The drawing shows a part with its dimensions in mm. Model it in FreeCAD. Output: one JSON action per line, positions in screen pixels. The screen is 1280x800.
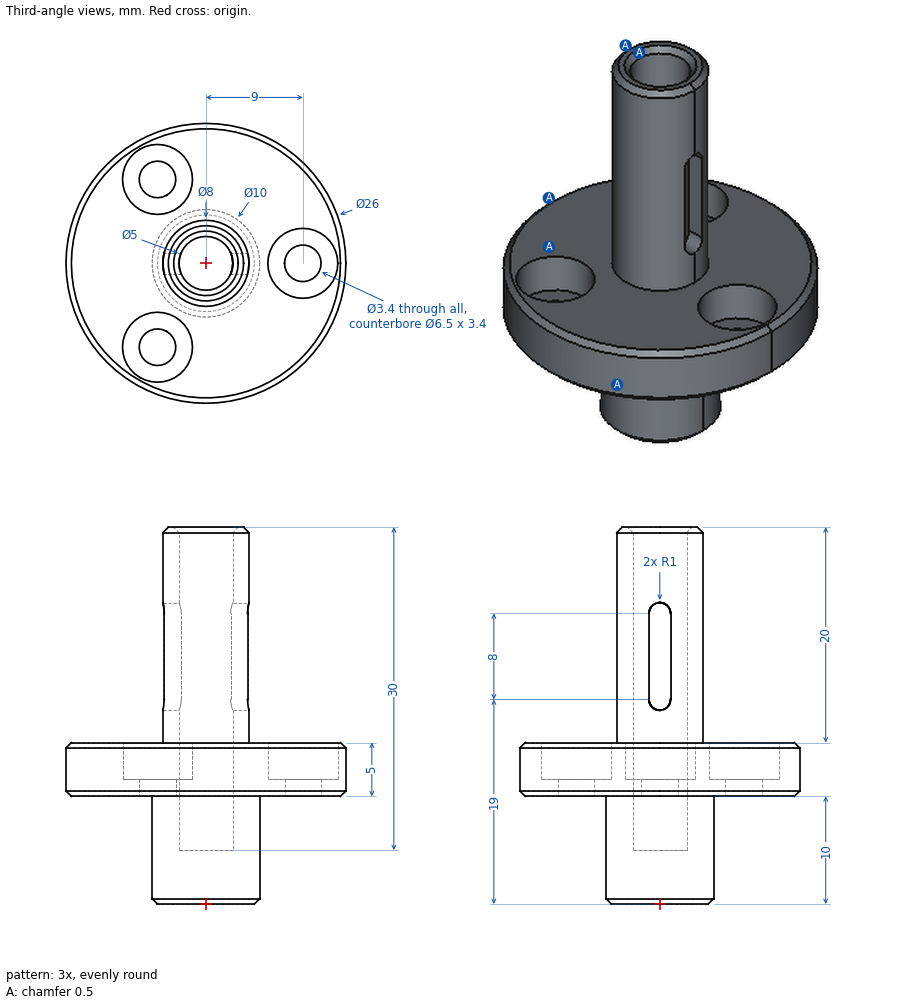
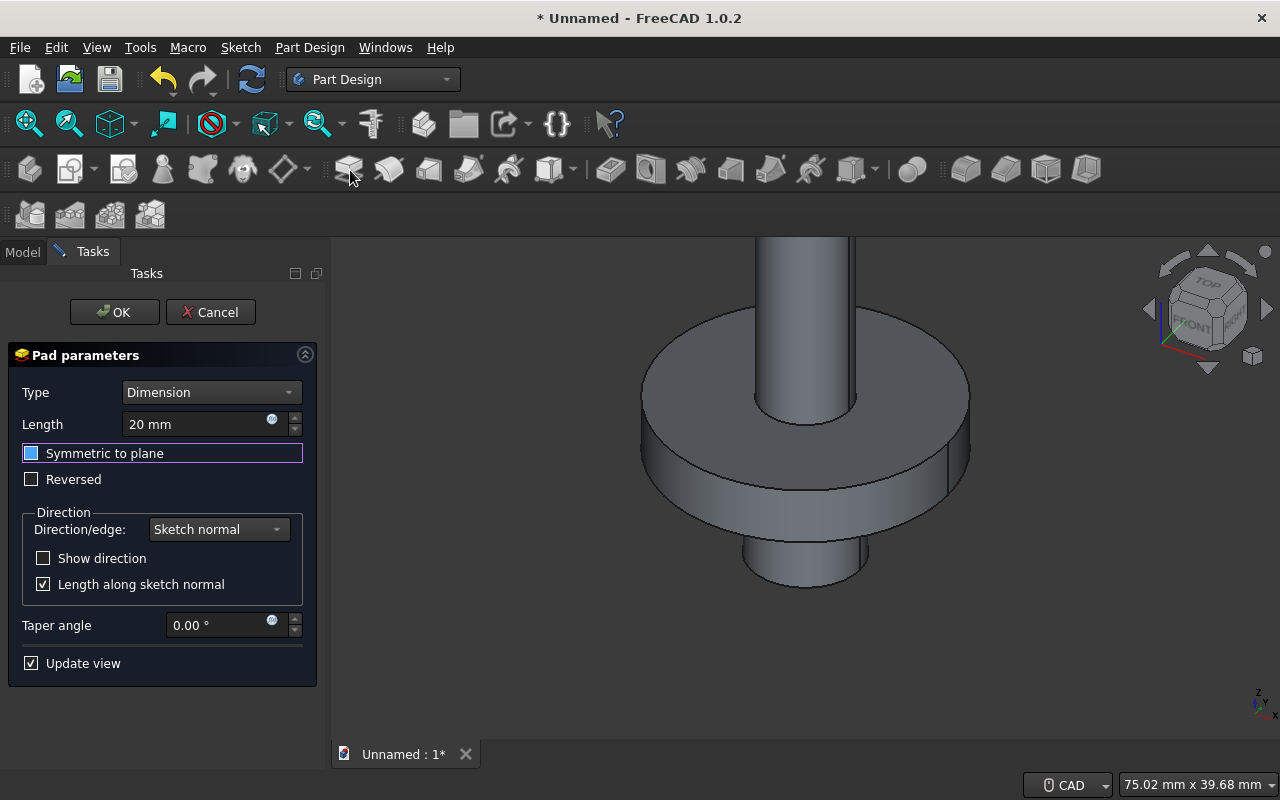
{"action": "left_click", "coordinate": [115, 312]}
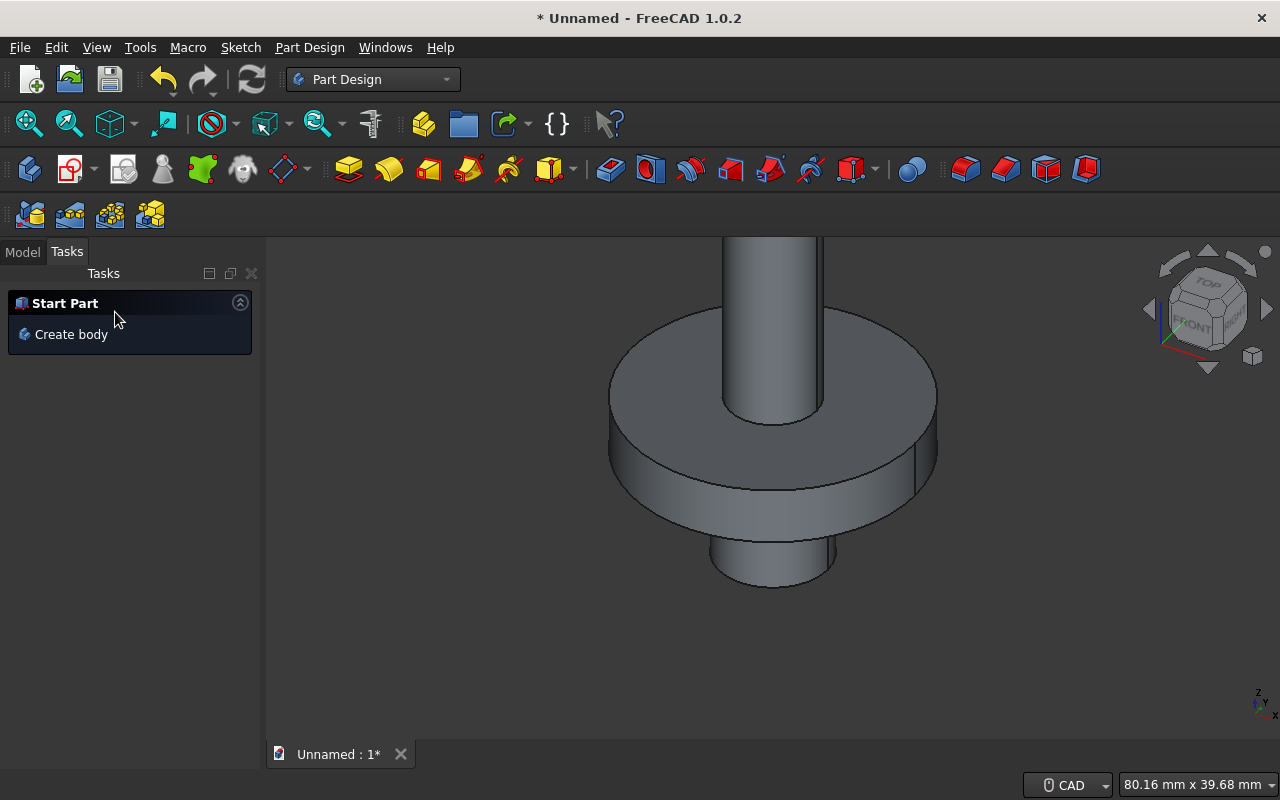
{"action": "left_click", "coordinate": [30, 124]}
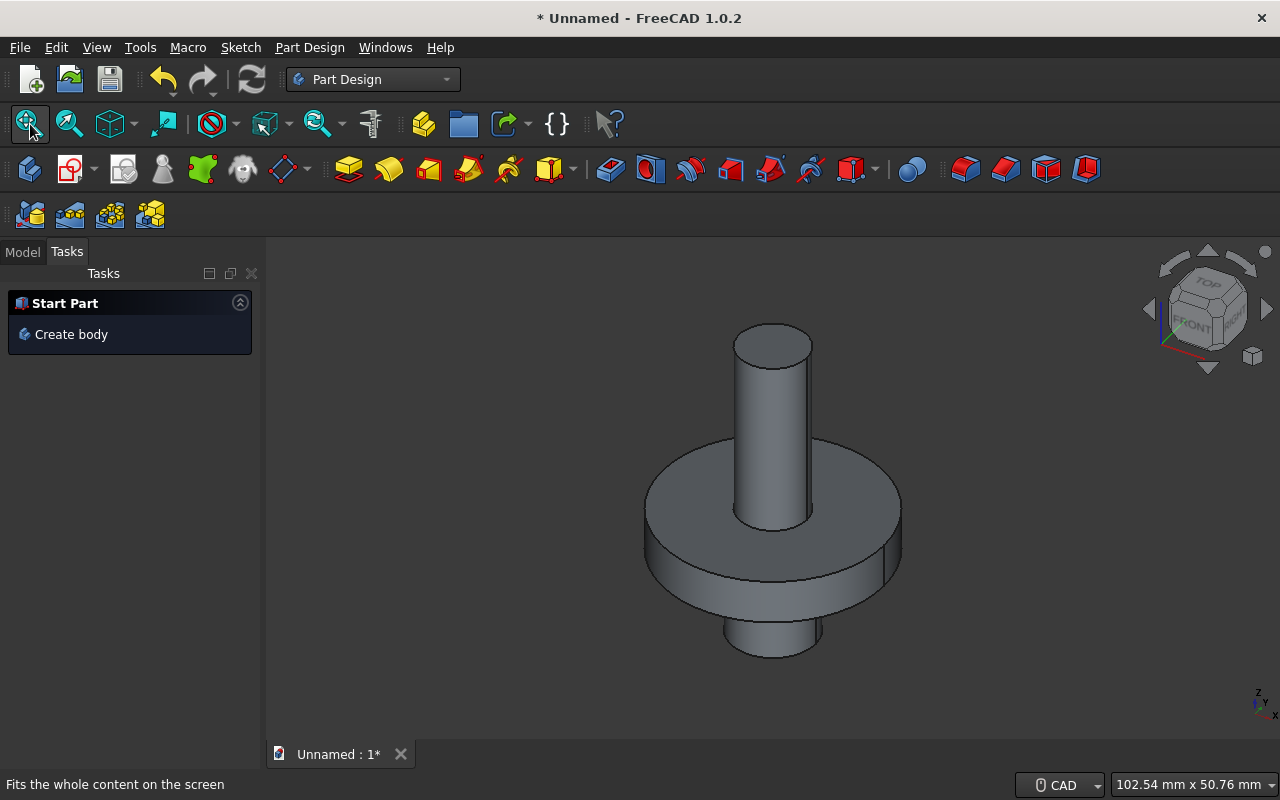
{"action": "left_click", "coordinate": [773, 345]}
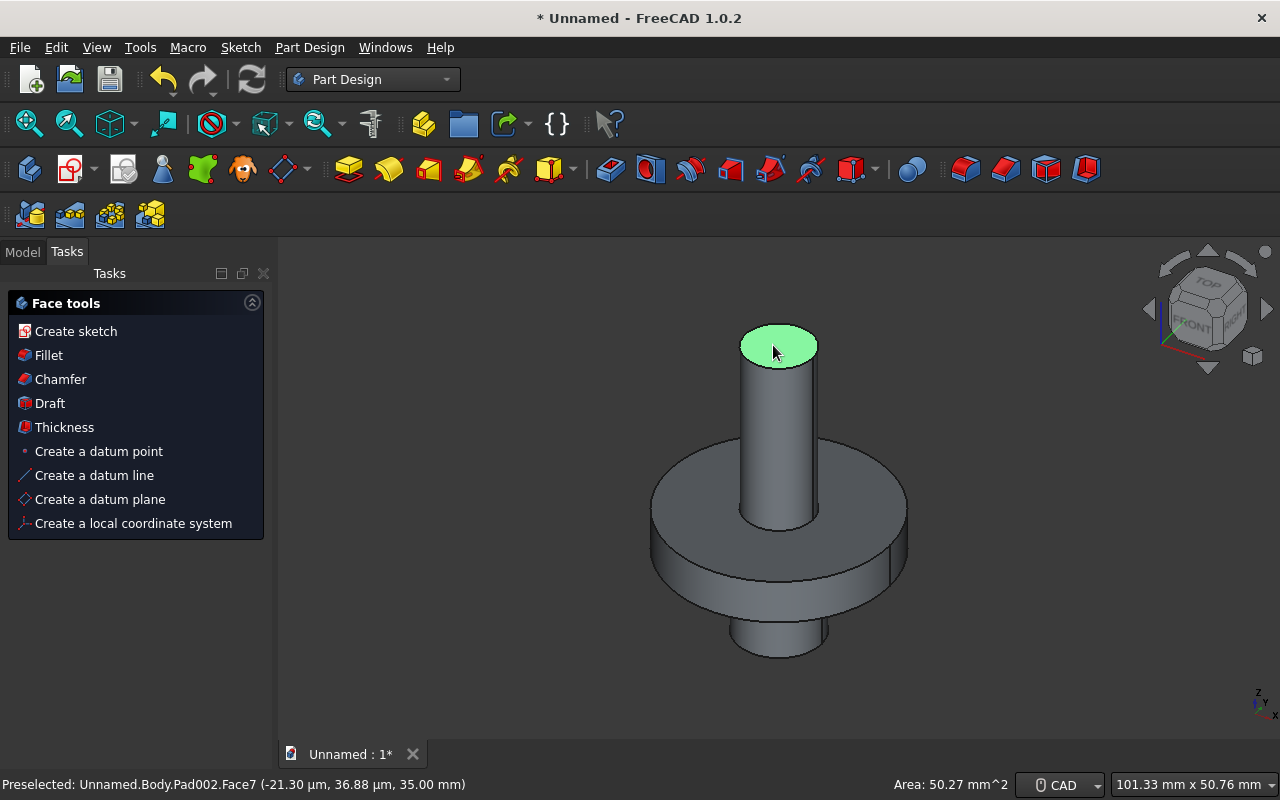
{"action": "left_click", "coordinate": [70, 170]}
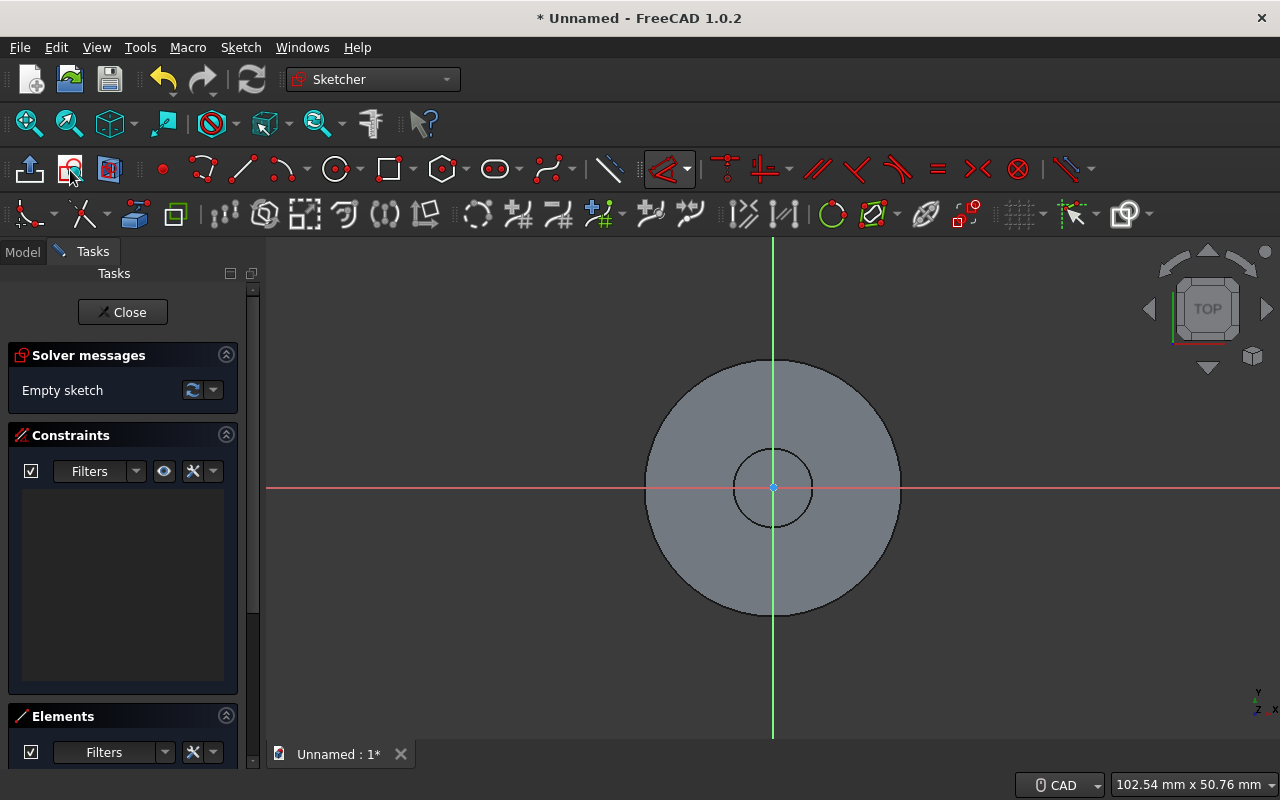
{"action": "scroll", "coordinate": [787, 488], "scroll_direction": "up", "scroll_amount": 9}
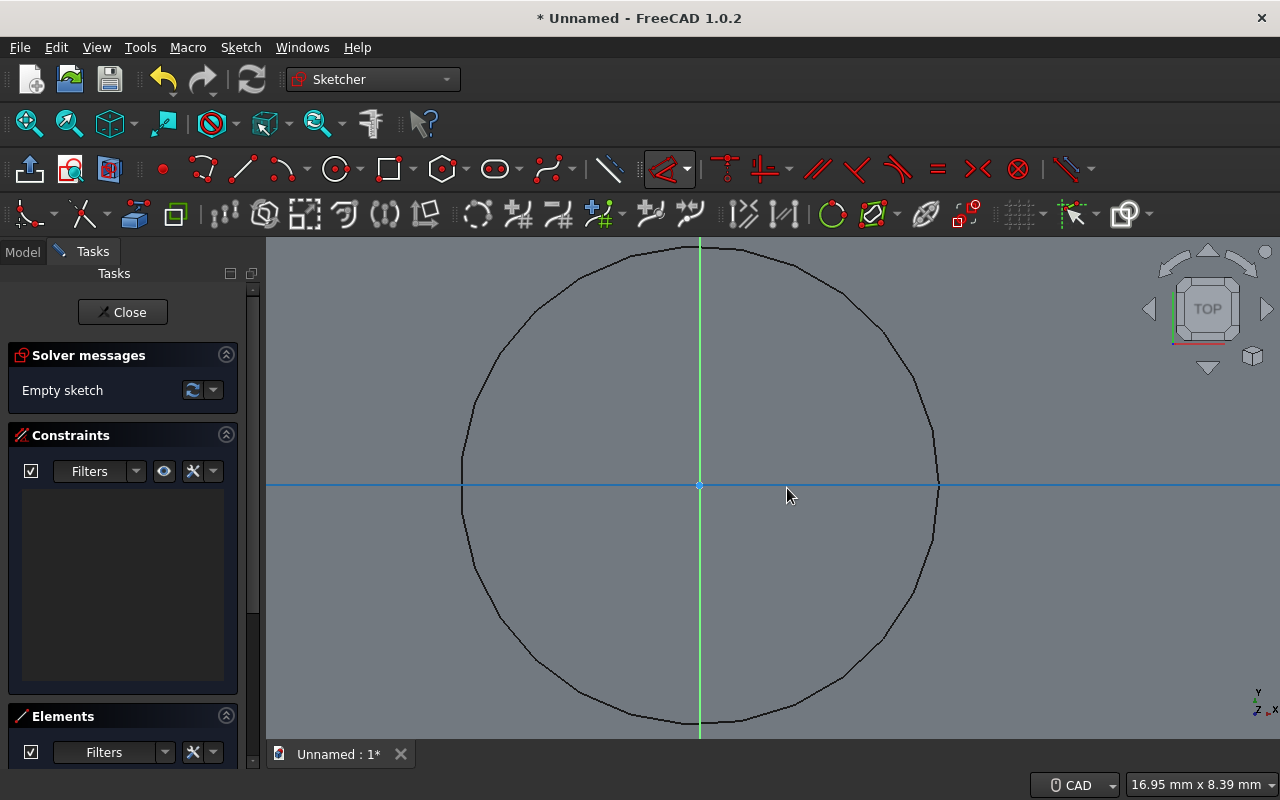
{"action": "left_click", "coordinate": [336, 170]}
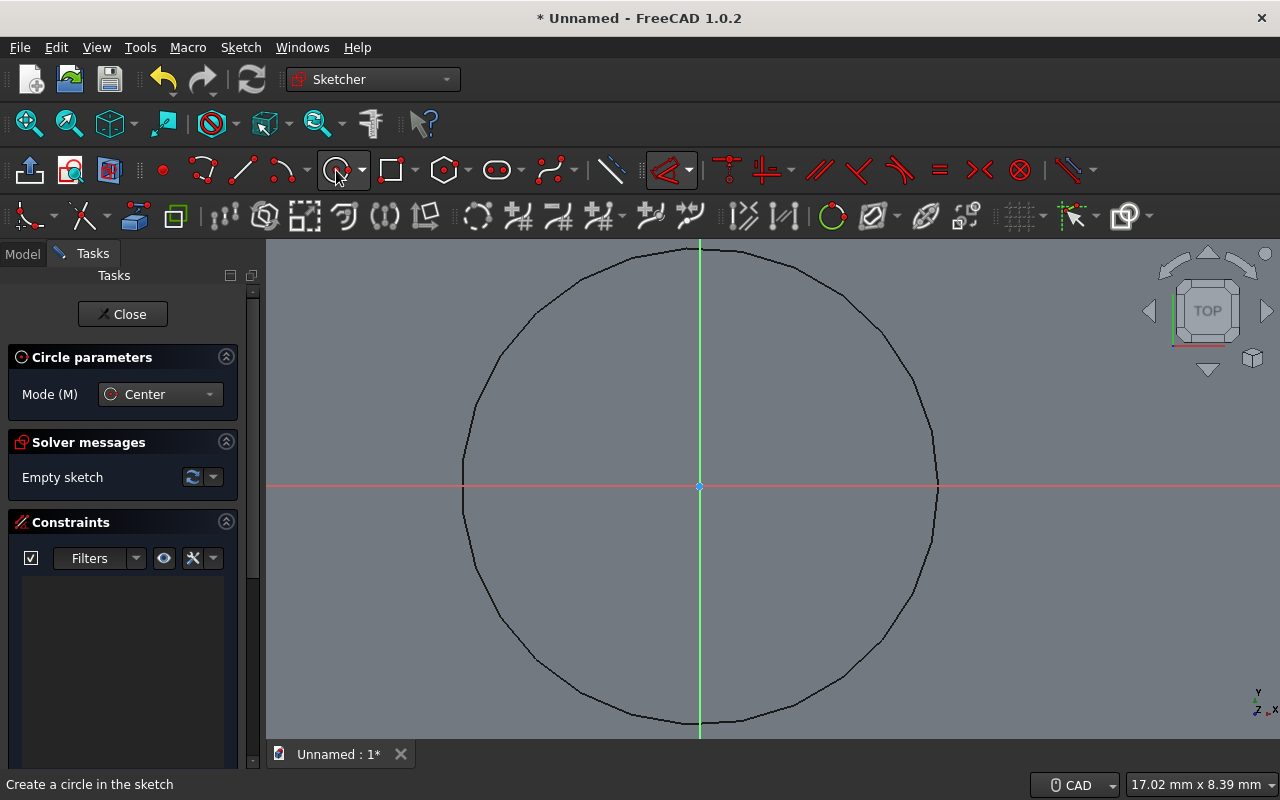
{"action": "left_click", "coordinate": [700, 486]}
{"action": "left_click", "coordinate": [805, 381]}
{"action": "key", "text": "Escape"}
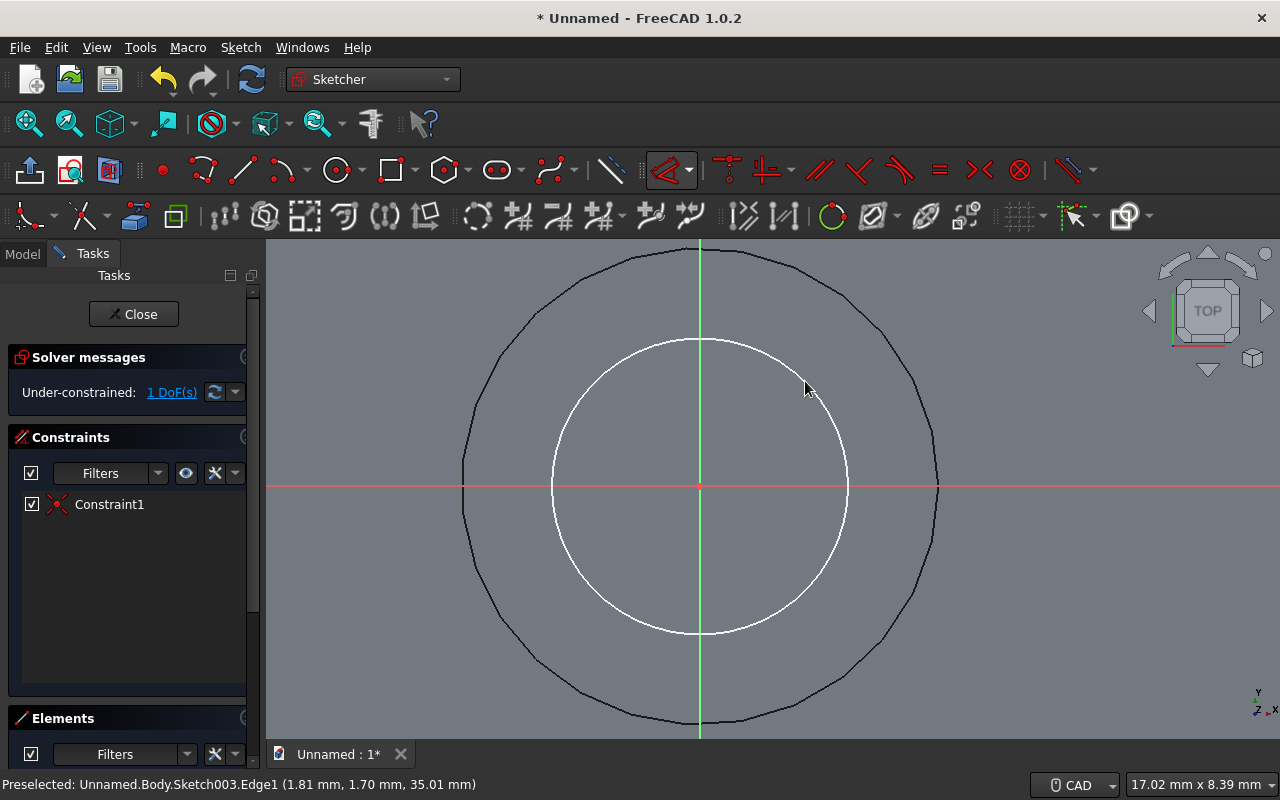
{"action": "left_click", "coordinate": [804, 381]}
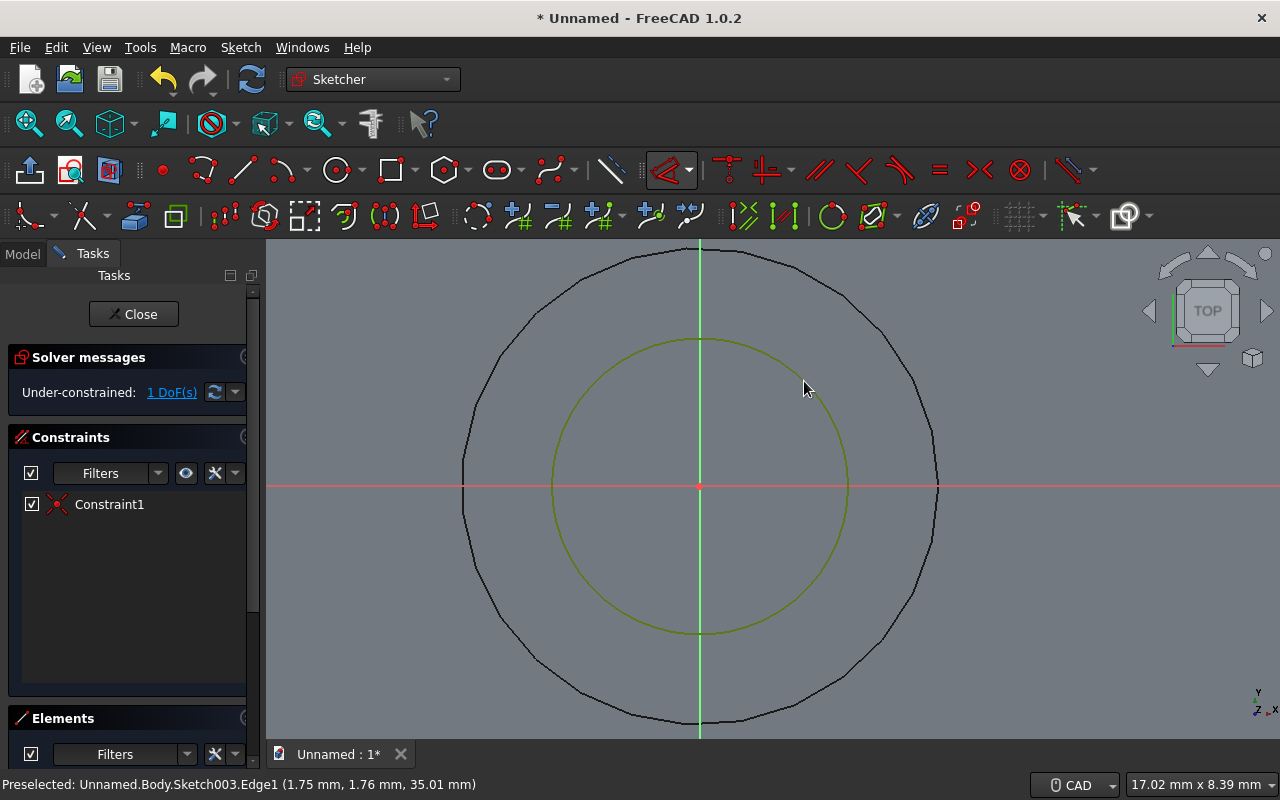
{"action": "left_click", "coordinate": [692, 170]}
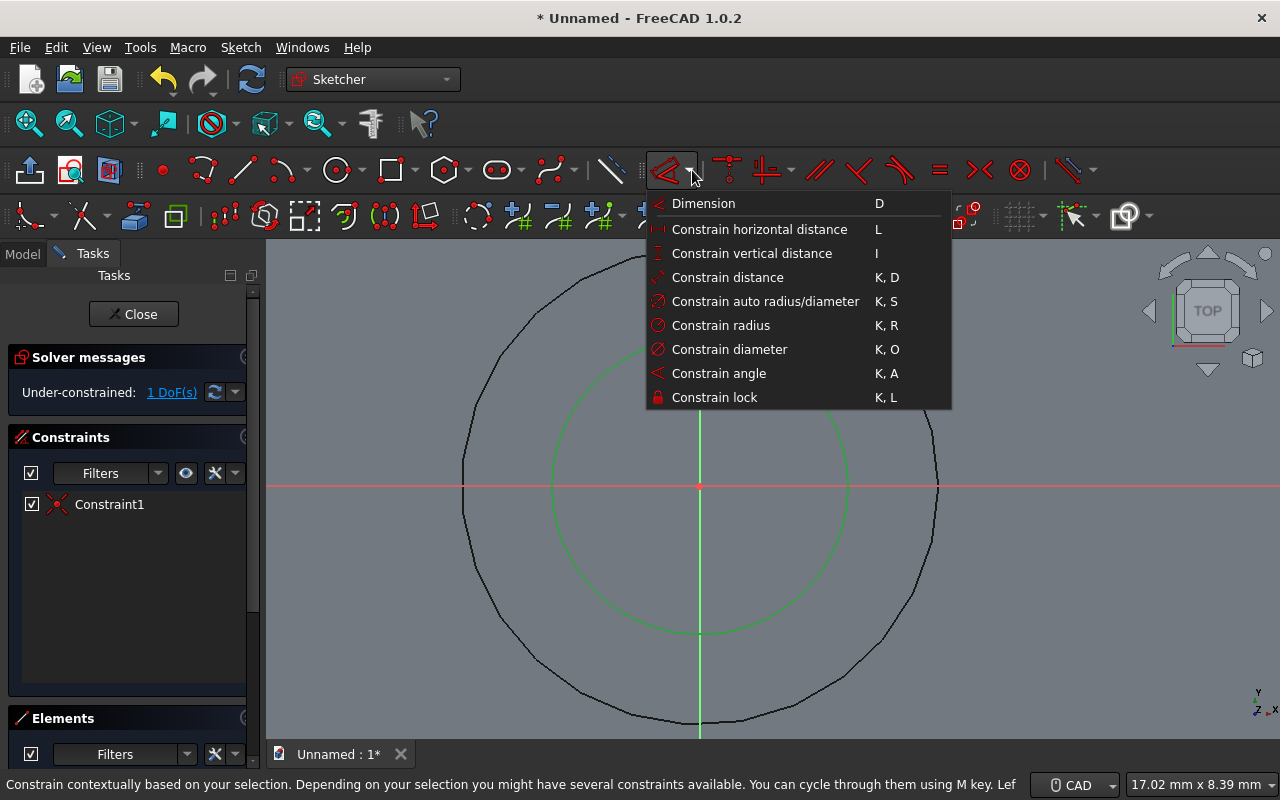
{"action": "left_click", "coordinate": [799, 349]}